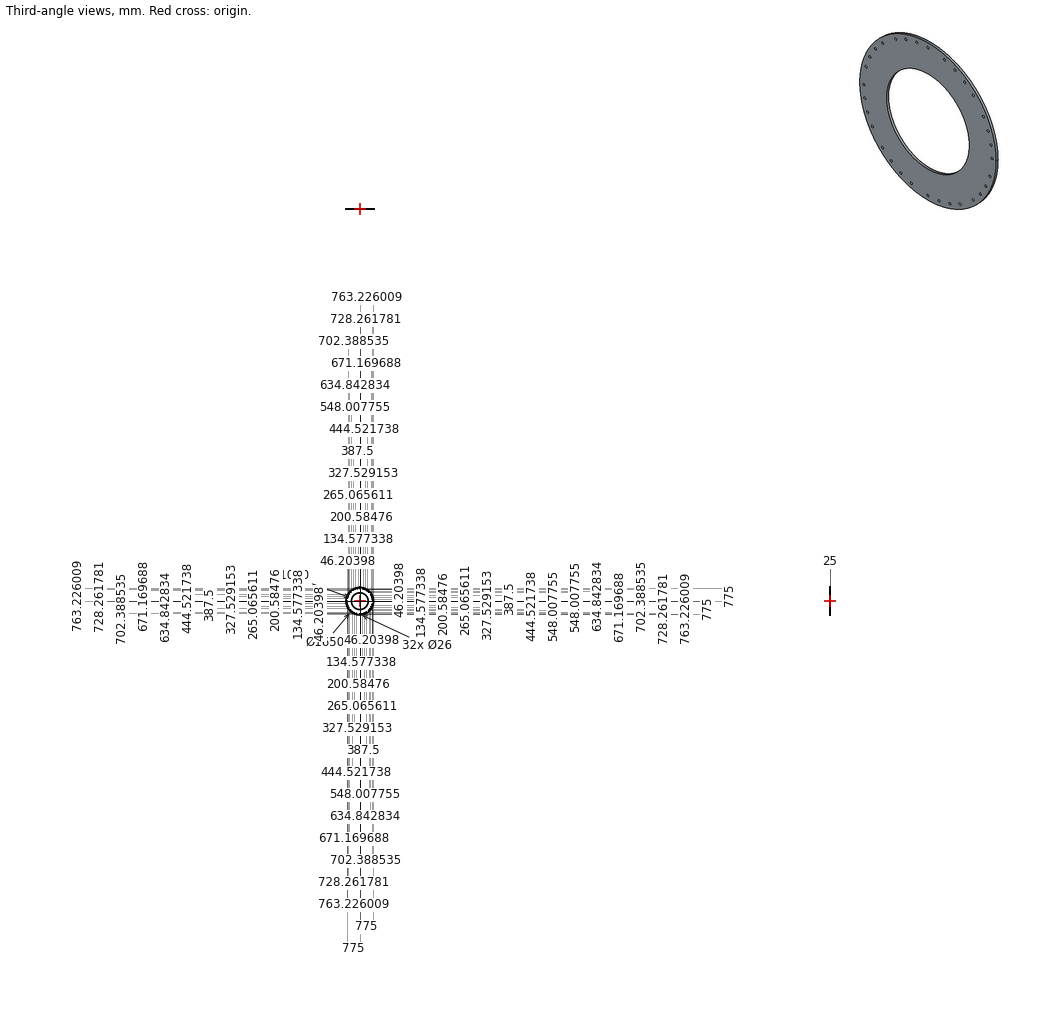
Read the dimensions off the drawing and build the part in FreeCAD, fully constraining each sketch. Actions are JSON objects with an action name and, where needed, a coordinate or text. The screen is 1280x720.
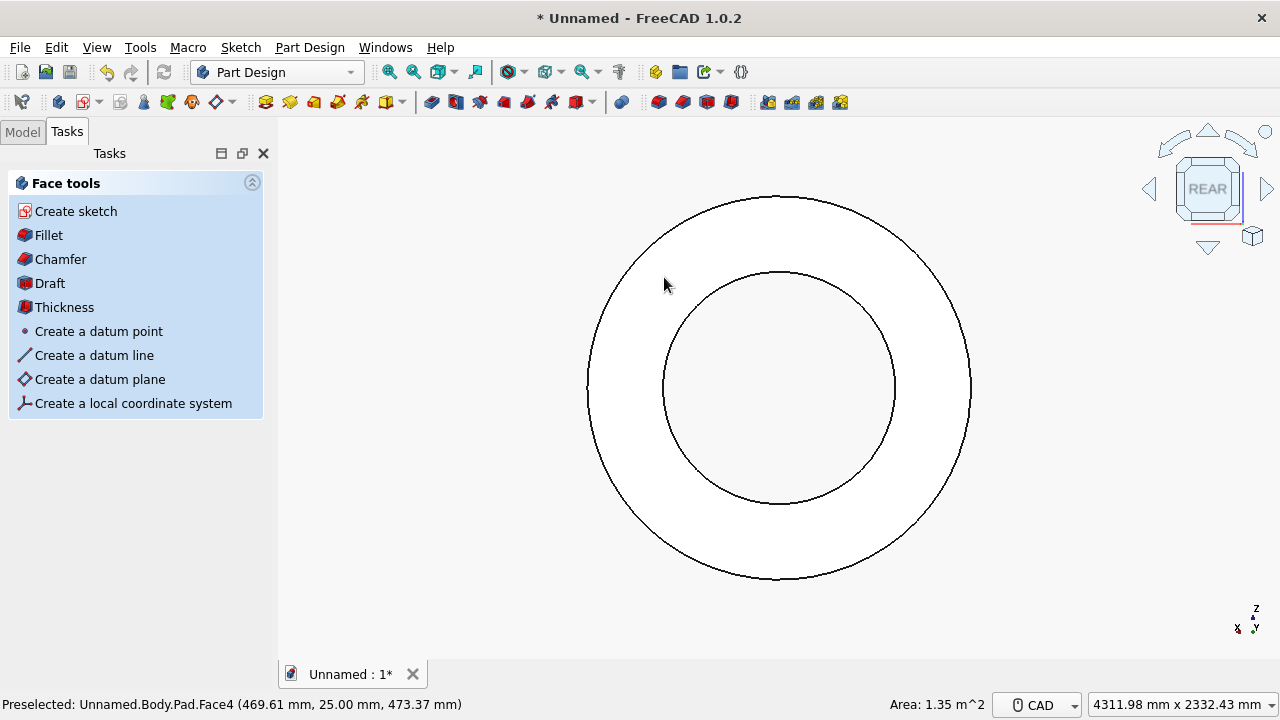
{"action": "left_click", "coordinate": [84, 102]}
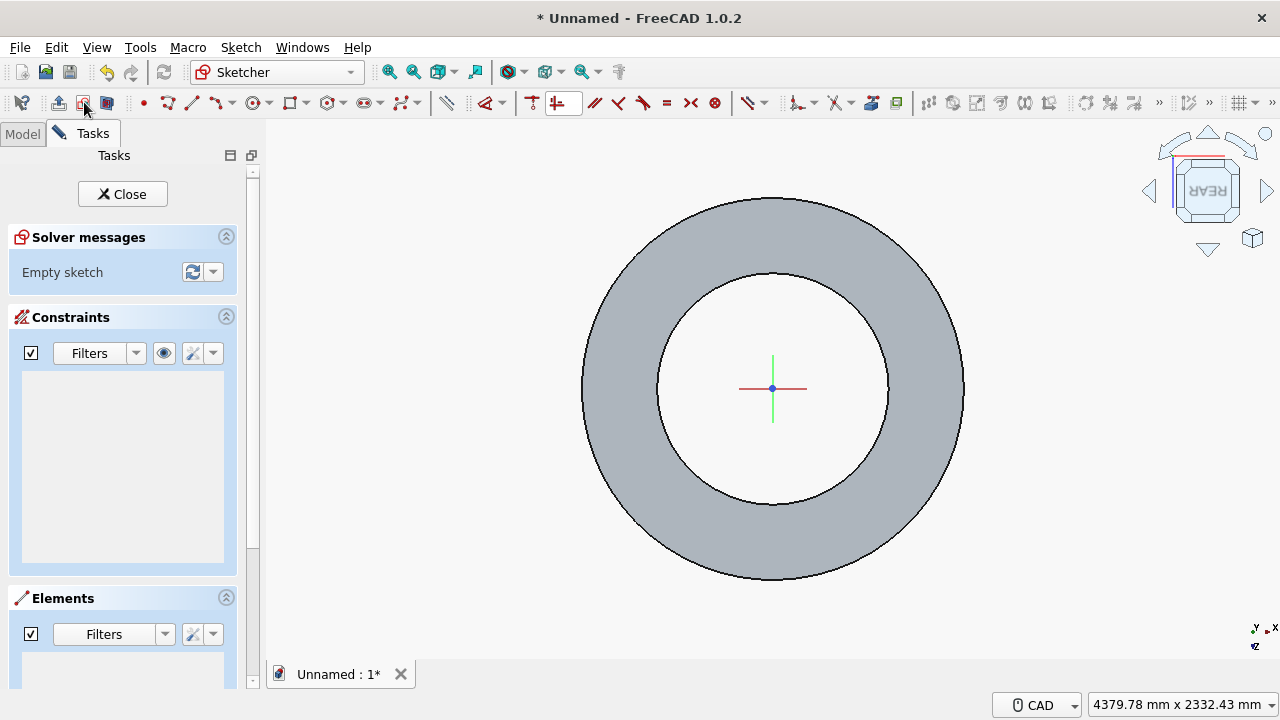
{"action": "left_click", "coordinate": [254, 104]}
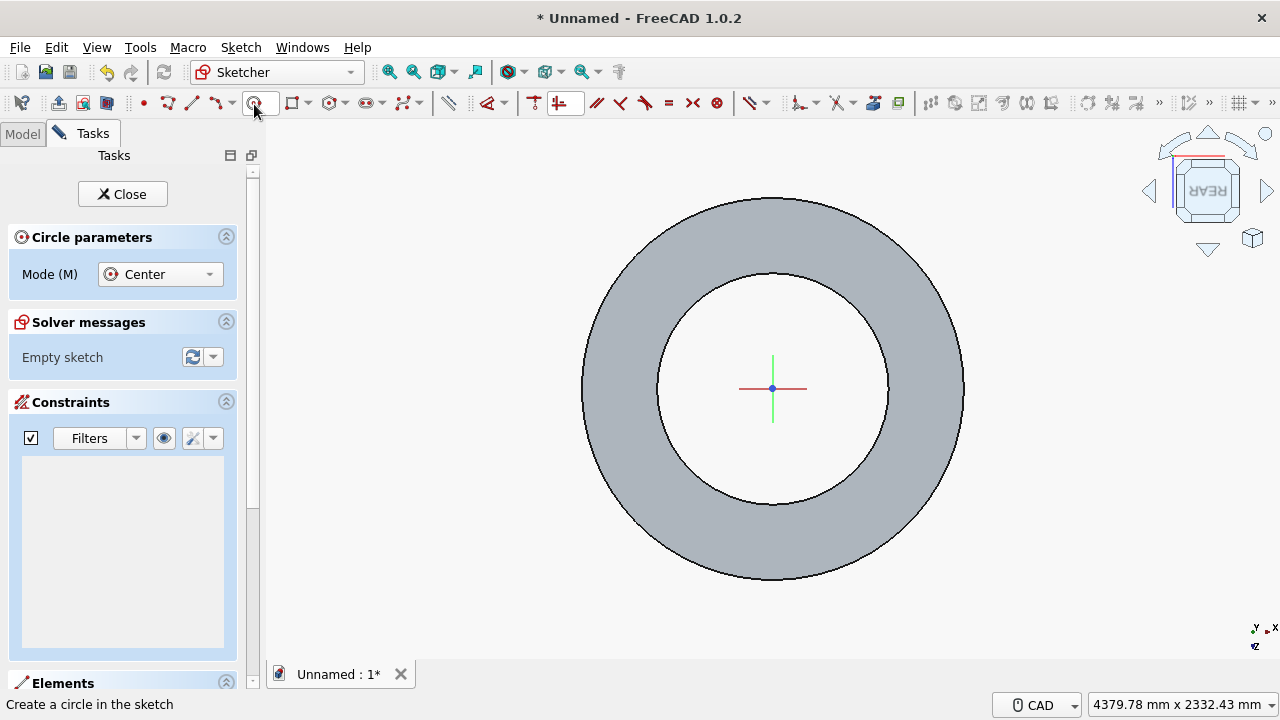
{"action": "scroll", "coordinate": [773, 210], "scroll_direction": "up", "scroll_amount": 11}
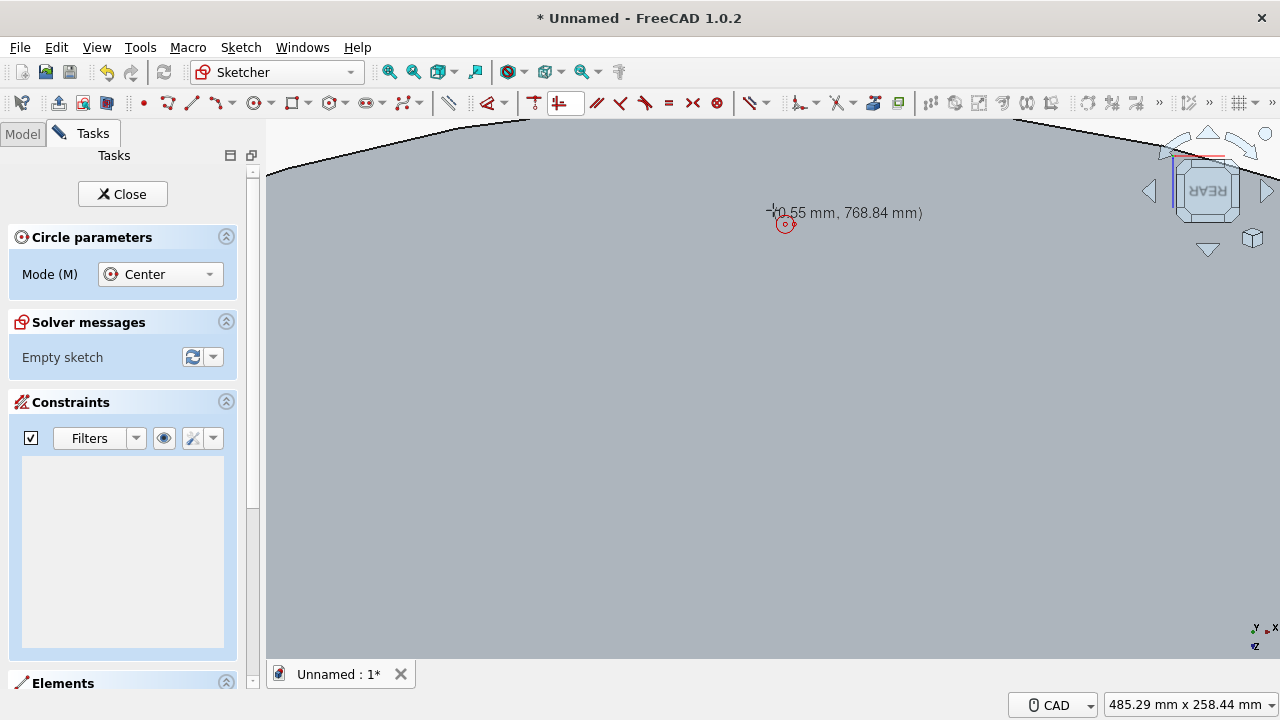
{"action": "scroll", "coordinate": [697, 210], "scroll_direction": "down", "scroll_amount": 11}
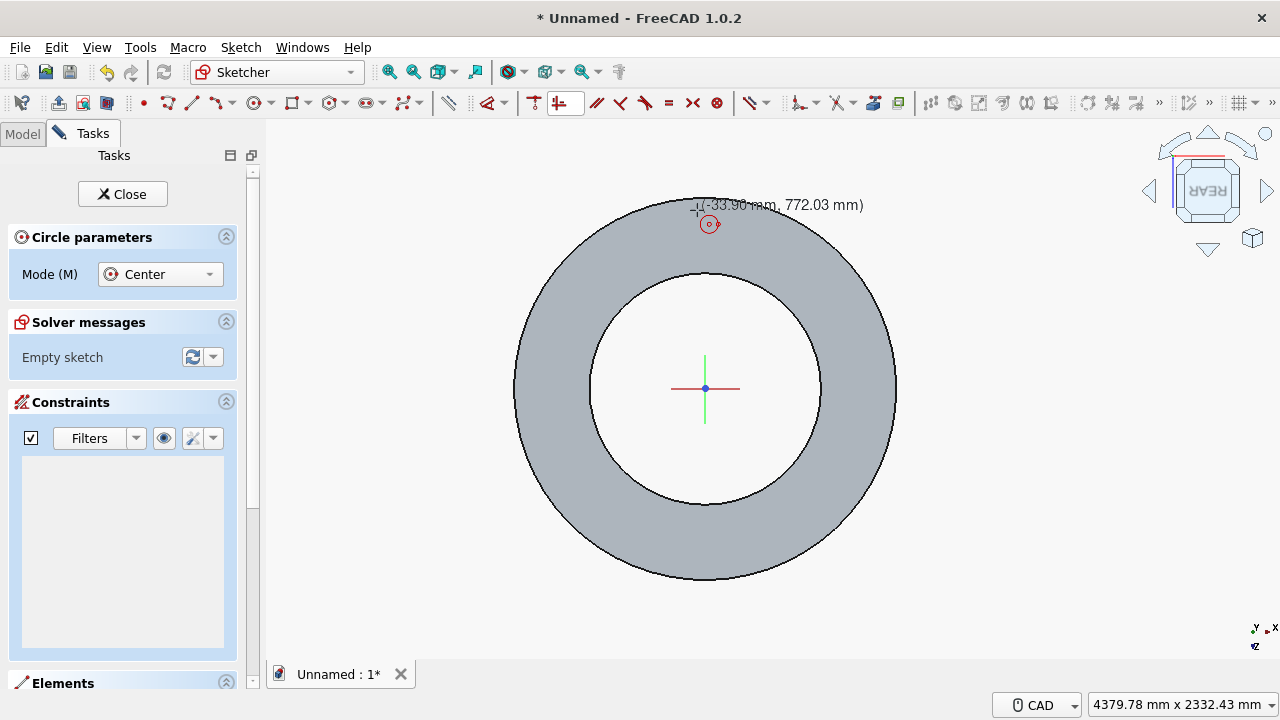
{"action": "left_click", "coordinate": [705, 210]}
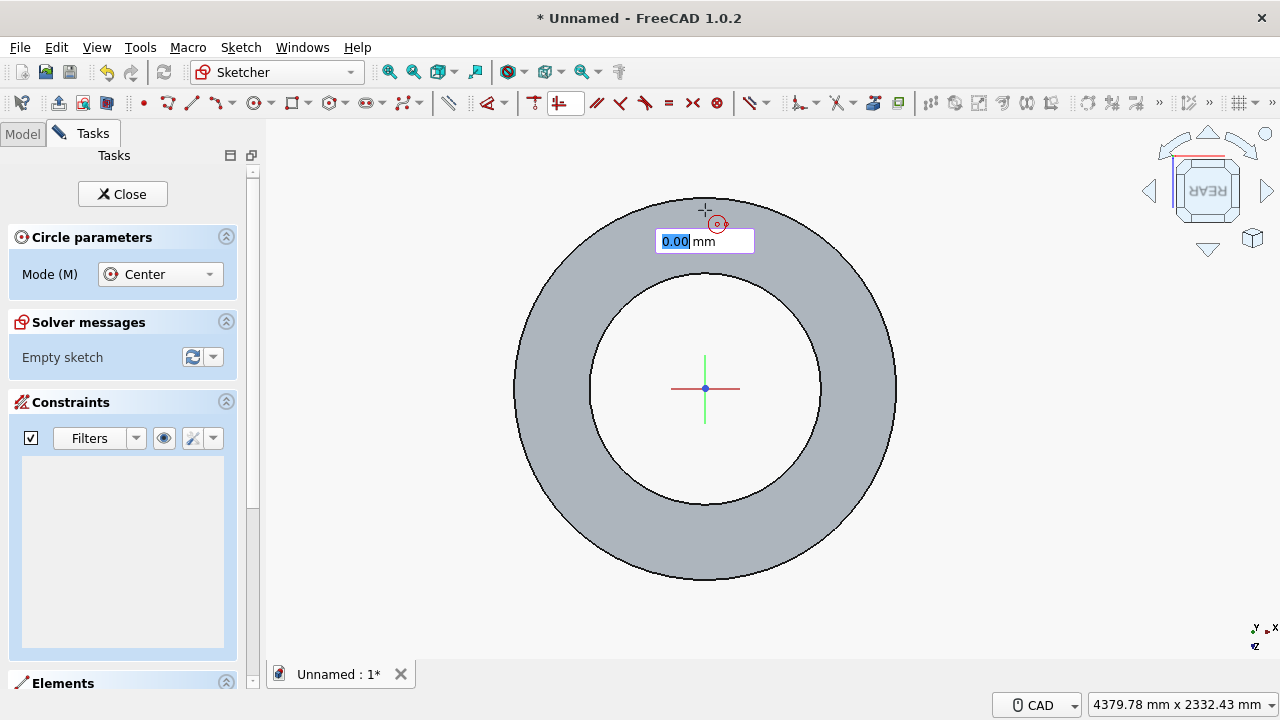
{"action": "scroll", "coordinate": [708, 209], "scroll_direction": "up", "scroll_amount": 9}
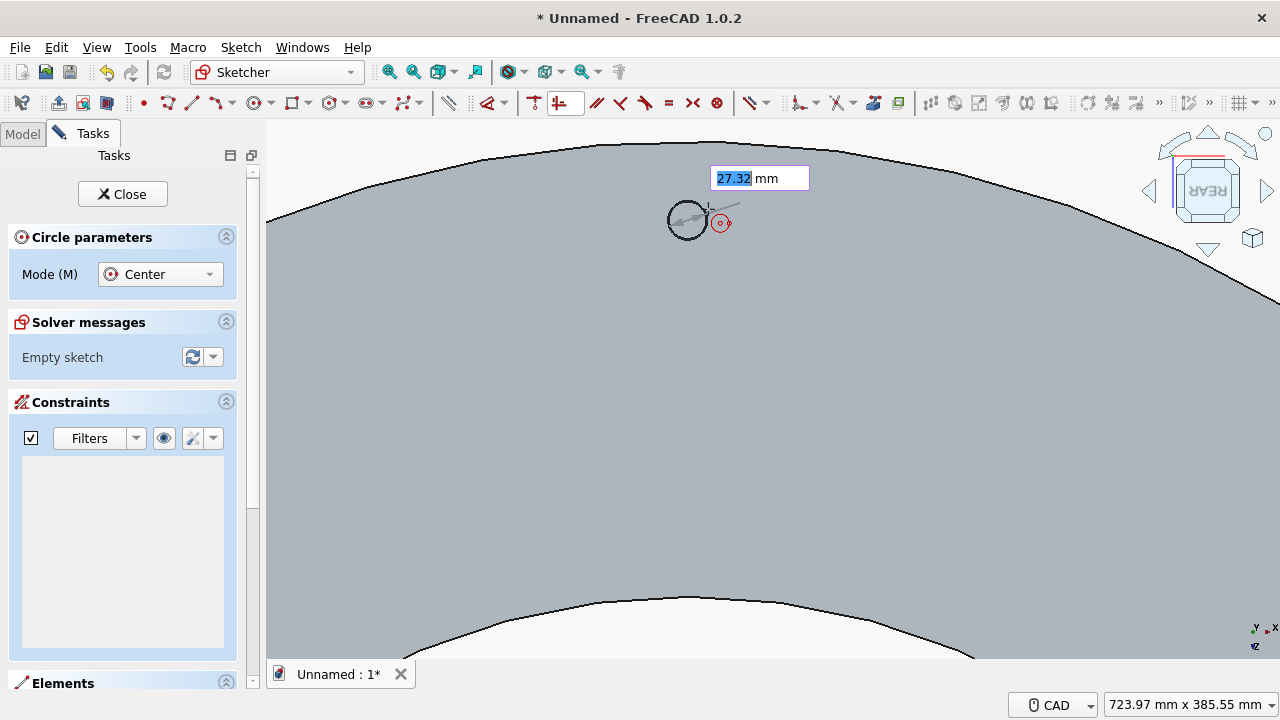
{"action": "left_click", "coordinate": [706, 205]}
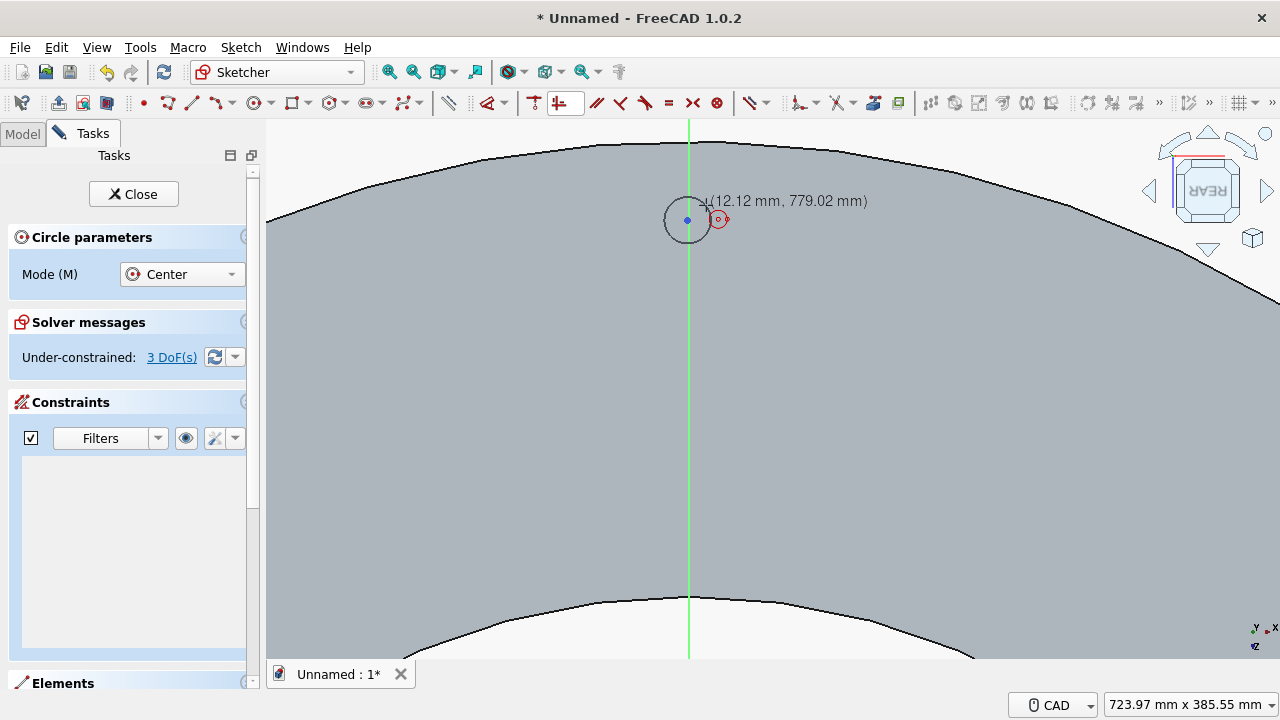
{"action": "scroll", "coordinate": [878, 228], "scroll_direction": "up", "scroll_amount": 2}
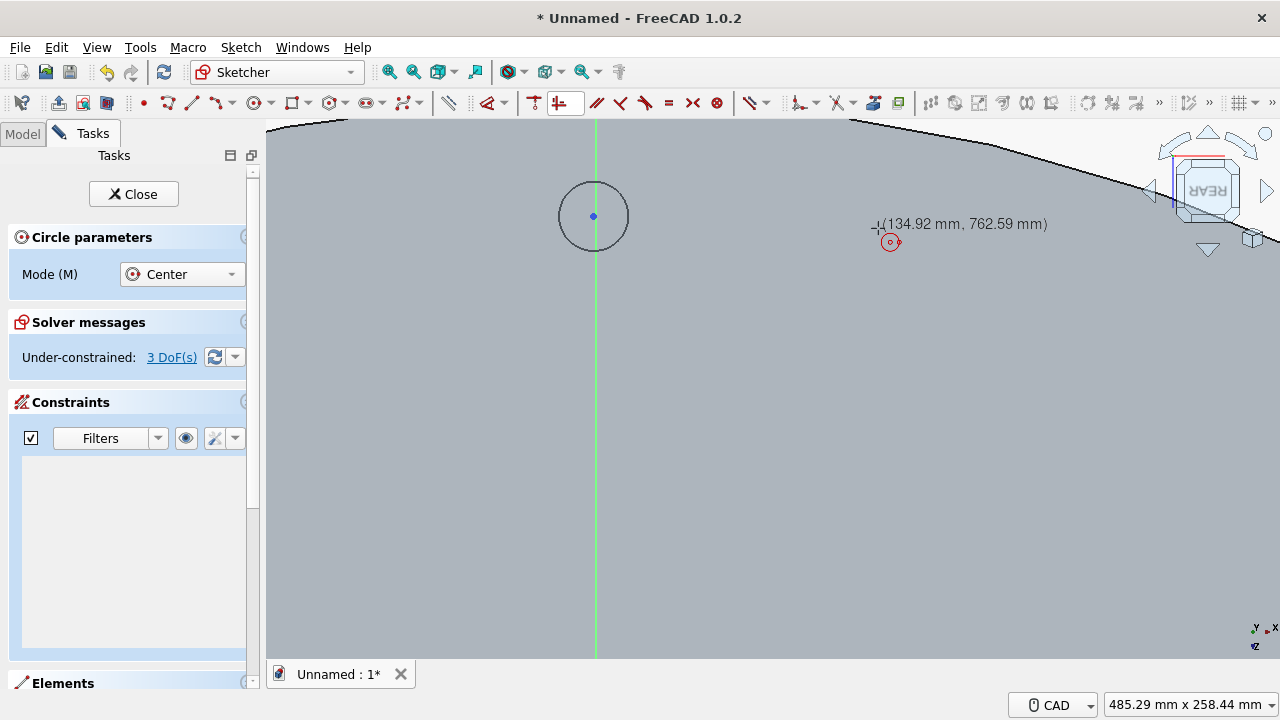
{"action": "scroll", "coordinate": [718, 210], "scroll_direction": "down", "scroll_amount": 11}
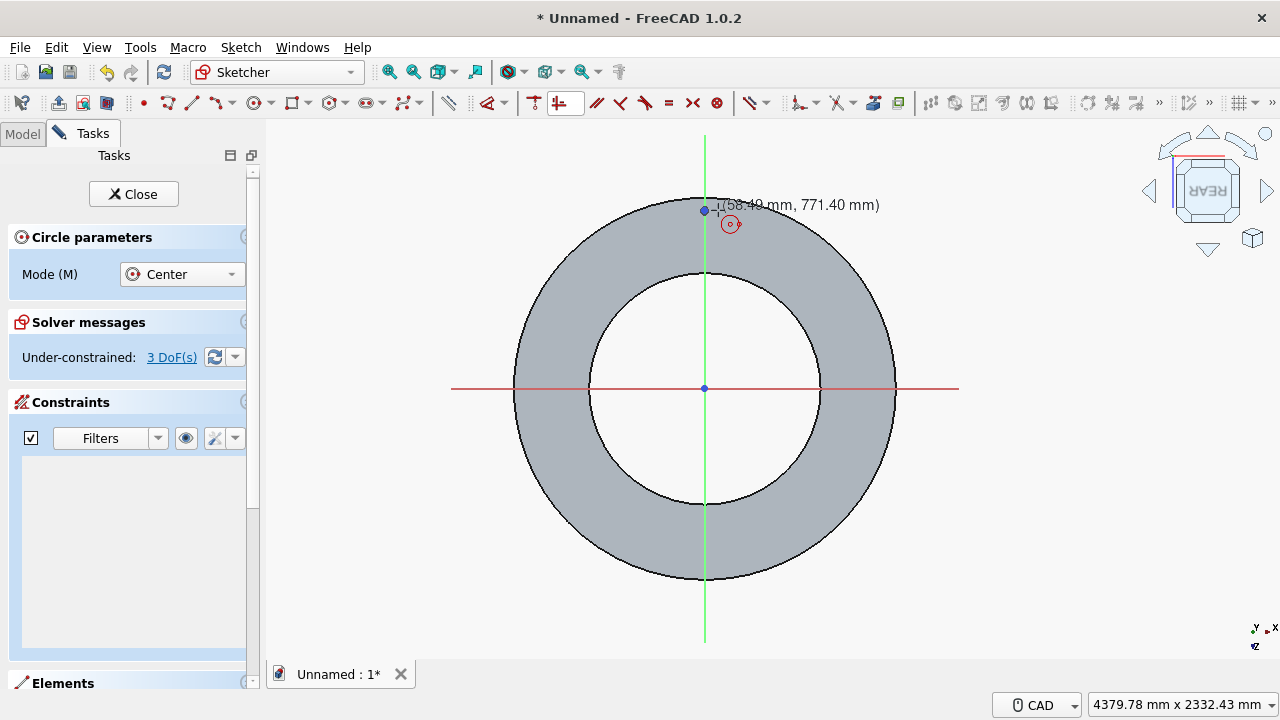
{"action": "left_click", "coordinate": [736, 212]}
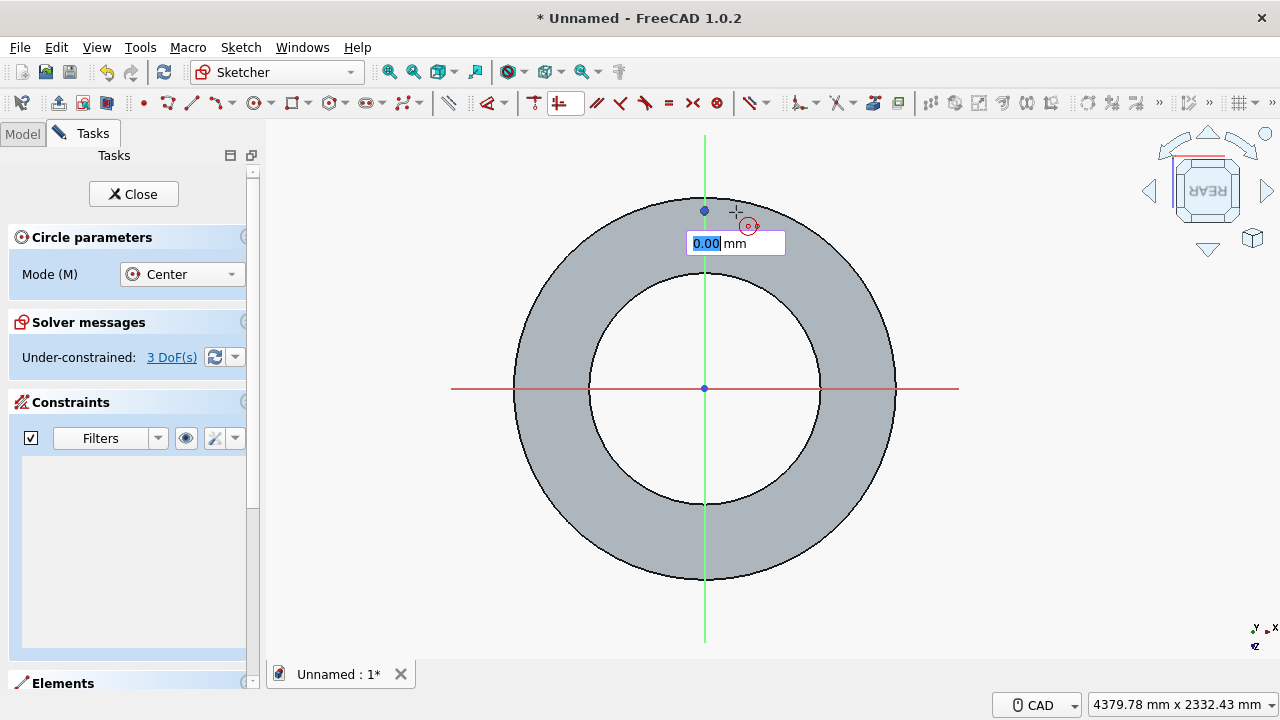
{"action": "scroll", "coordinate": [738, 210], "scroll_direction": "up", "scroll_amount": 9}